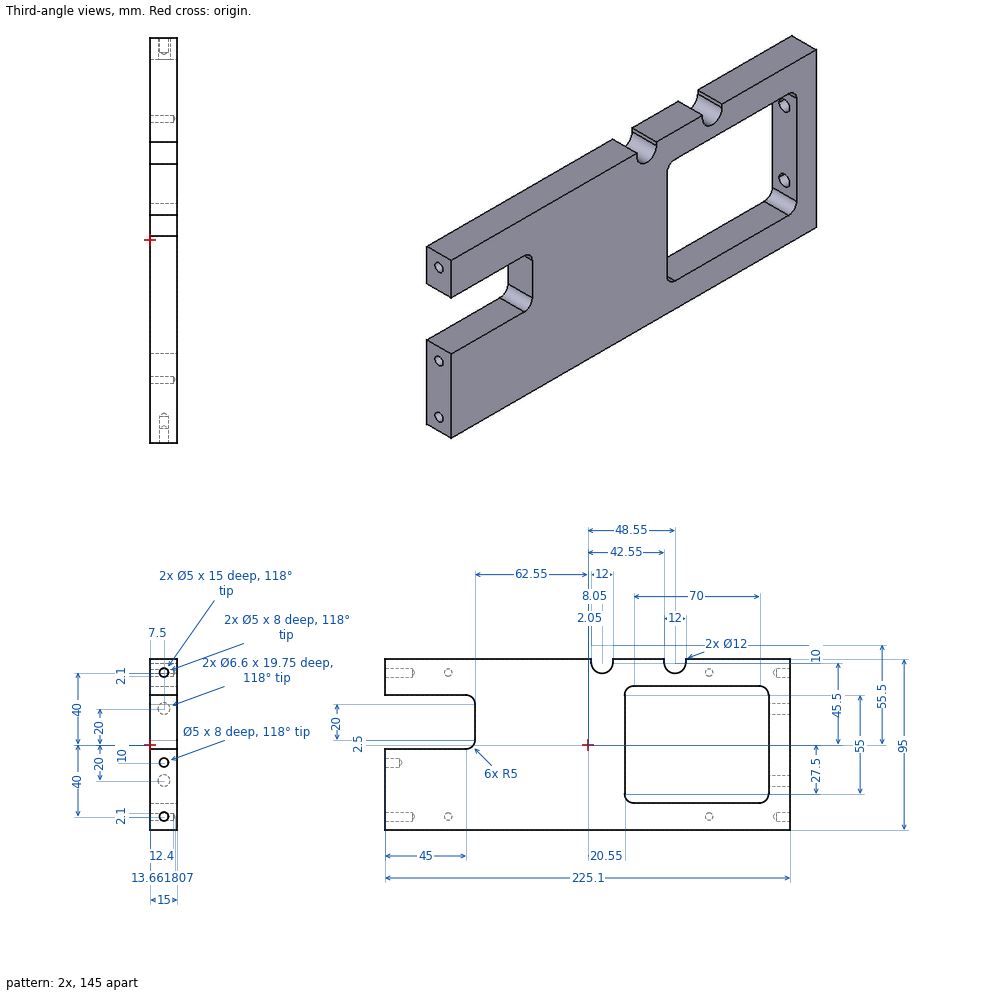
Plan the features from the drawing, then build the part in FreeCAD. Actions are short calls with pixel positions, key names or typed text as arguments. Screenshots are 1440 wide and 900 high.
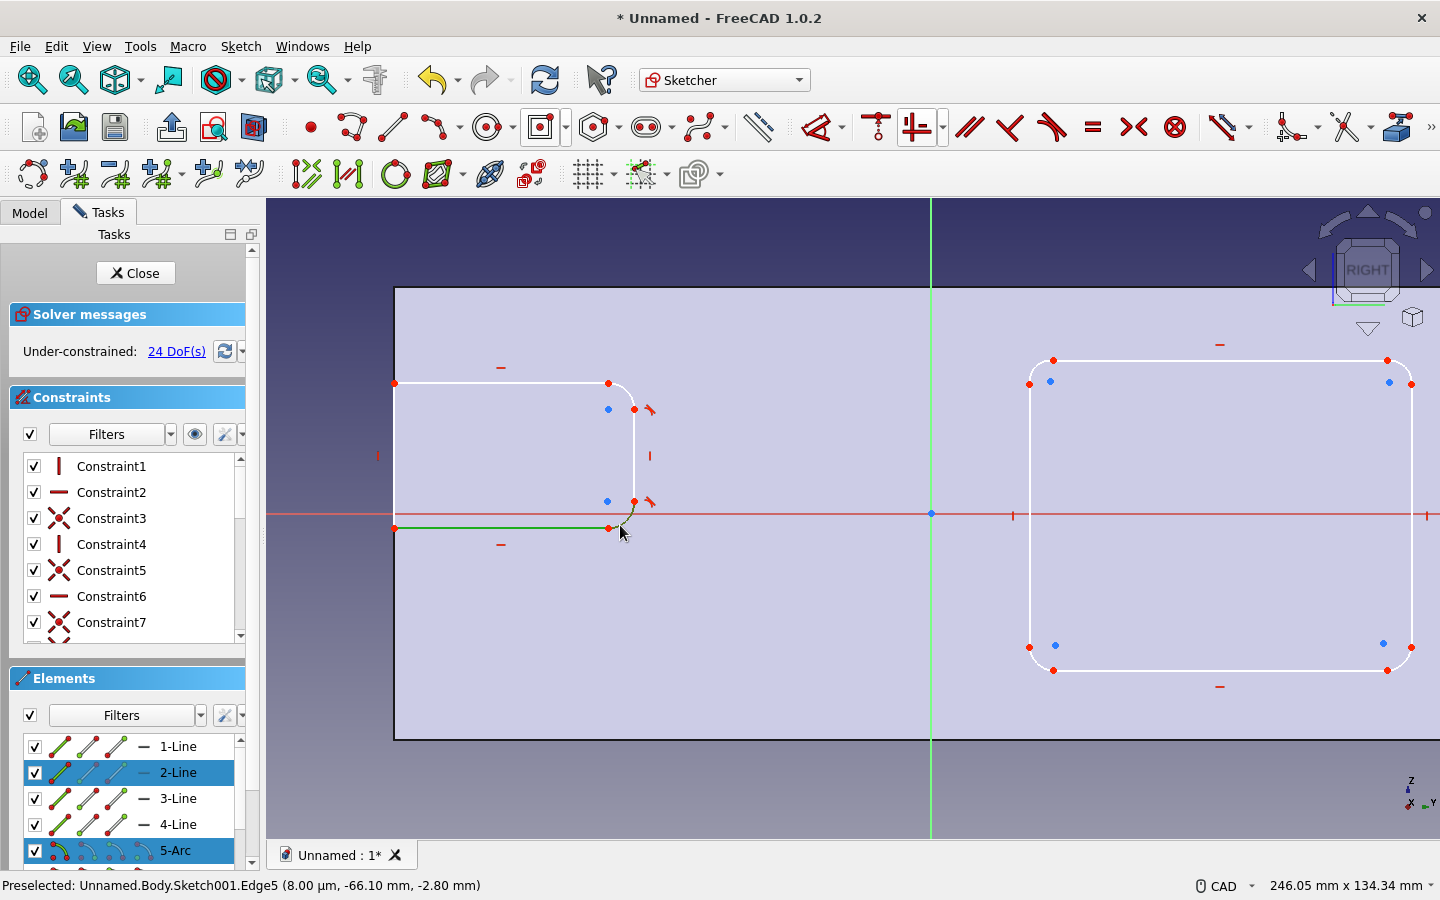
click(1052, 128)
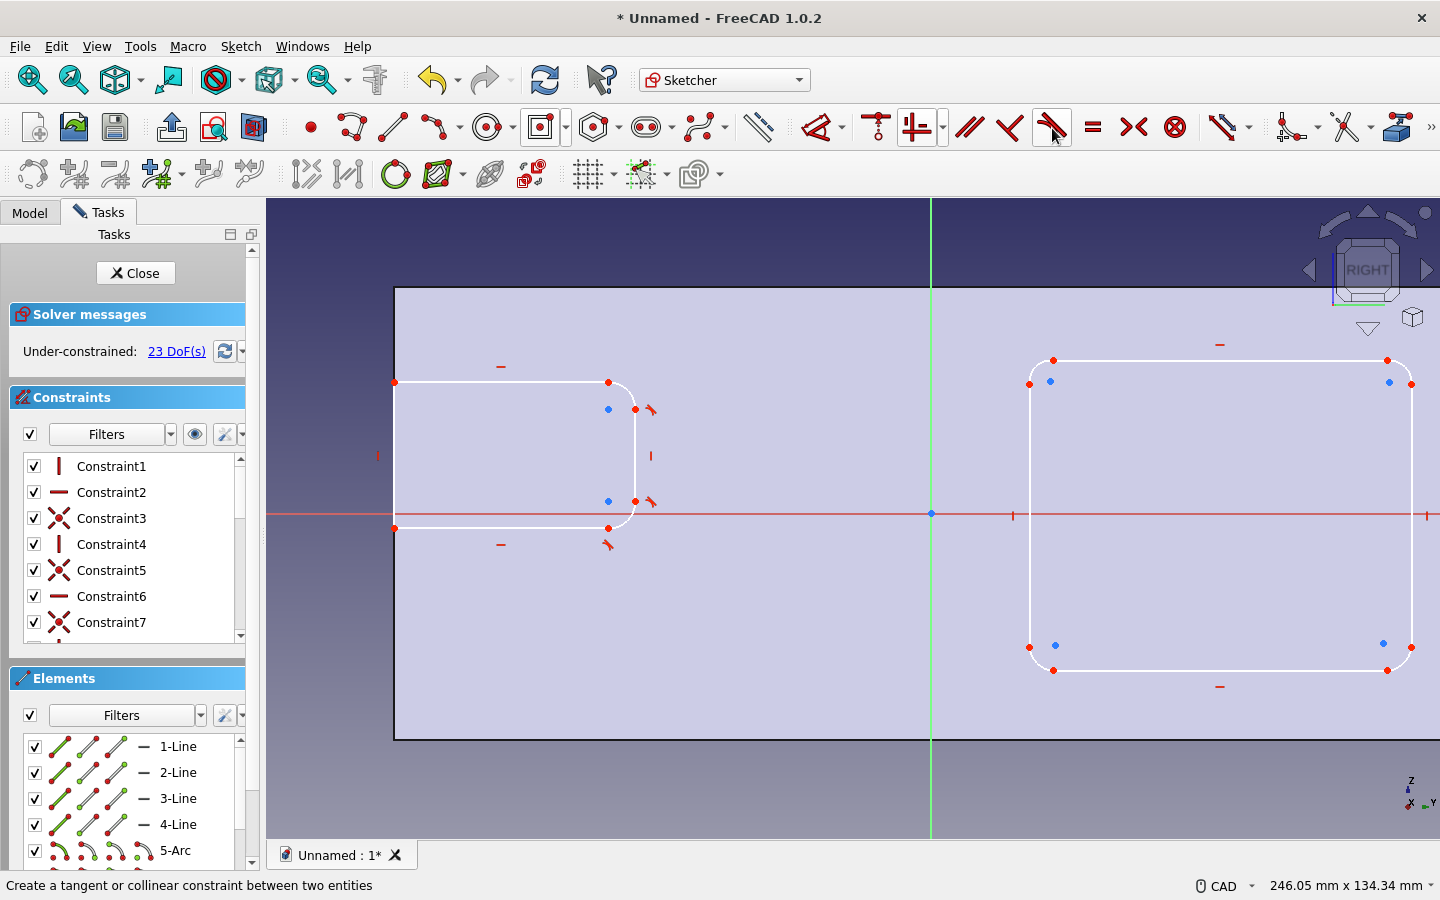
click(459, 382)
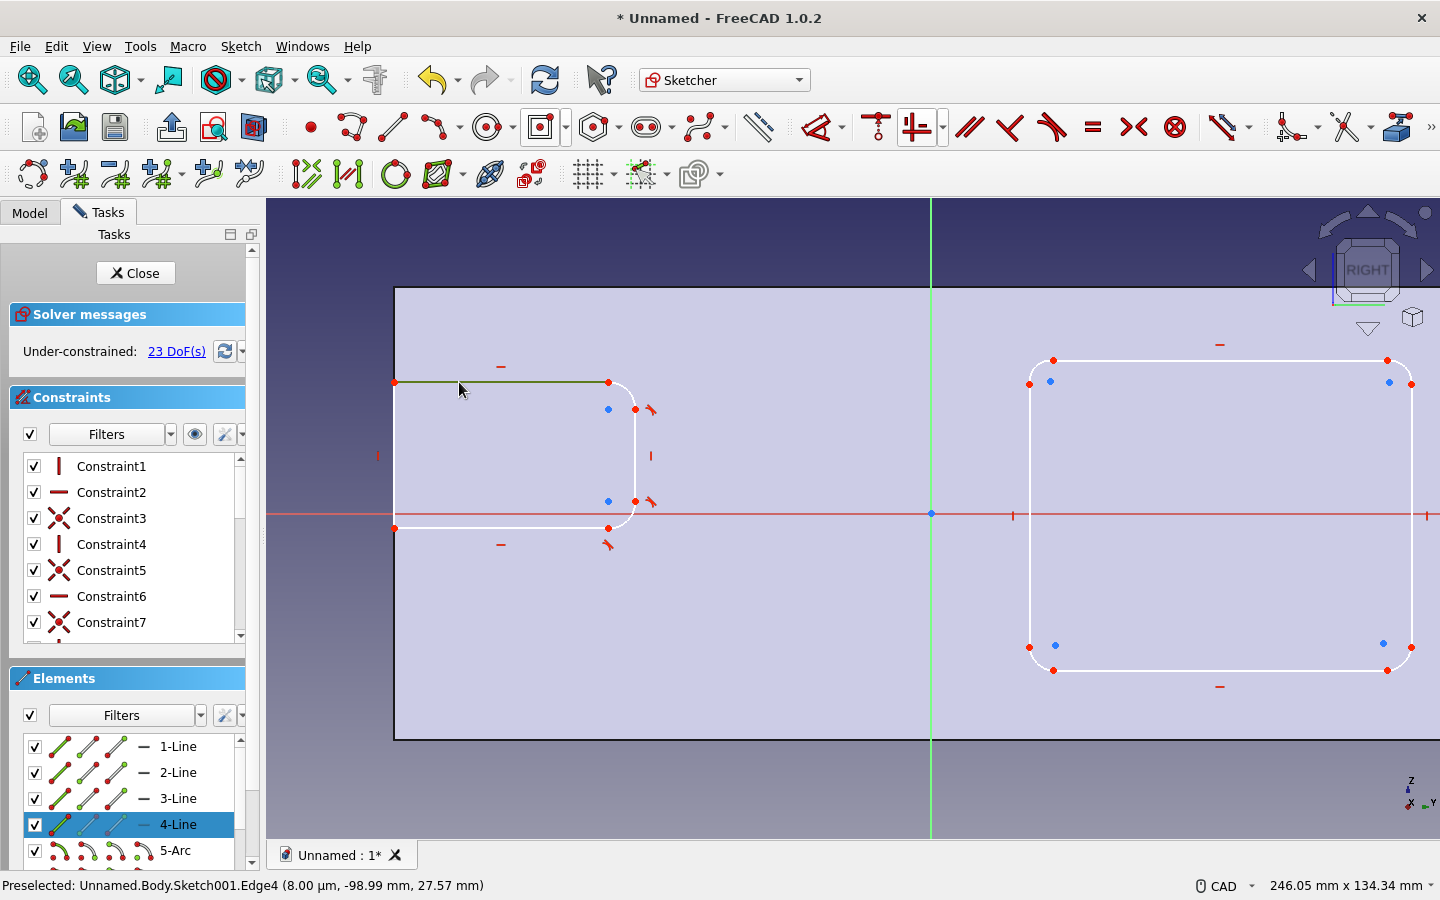
click(632, 397)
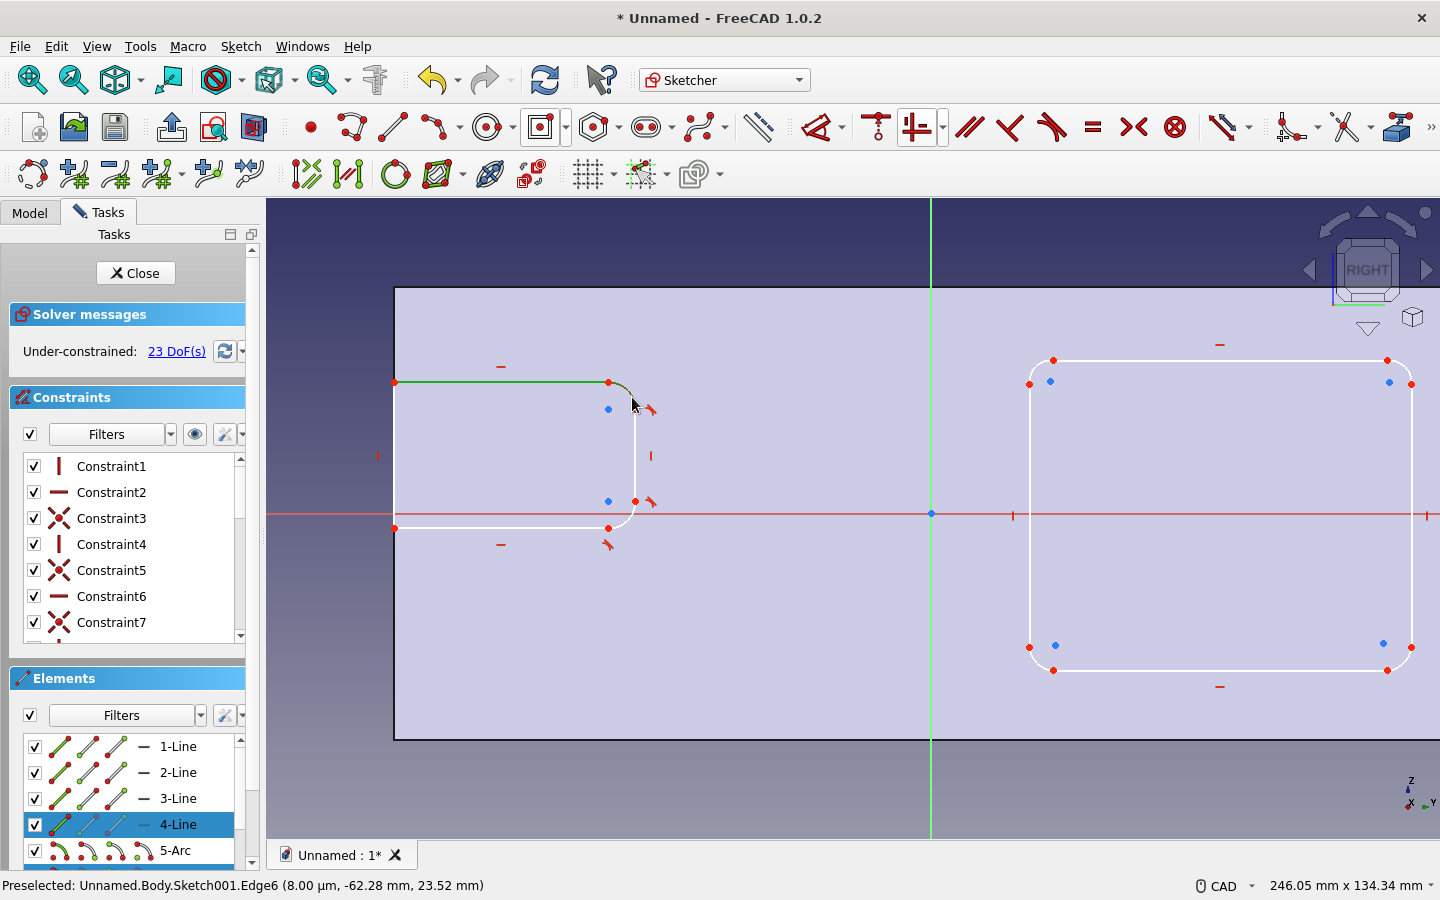
click(1052, 128)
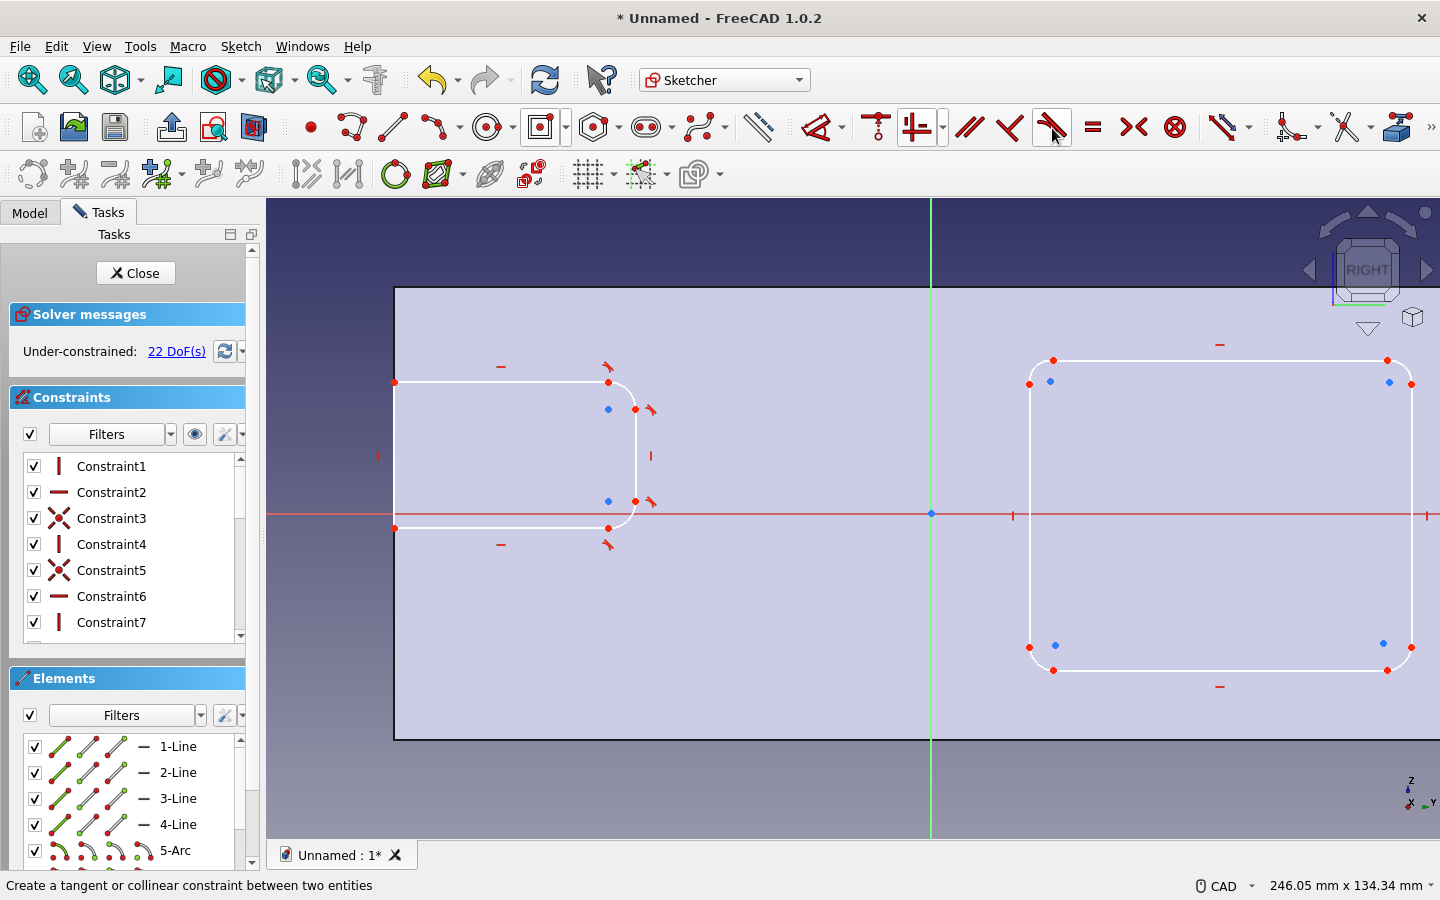
click(1030, 568)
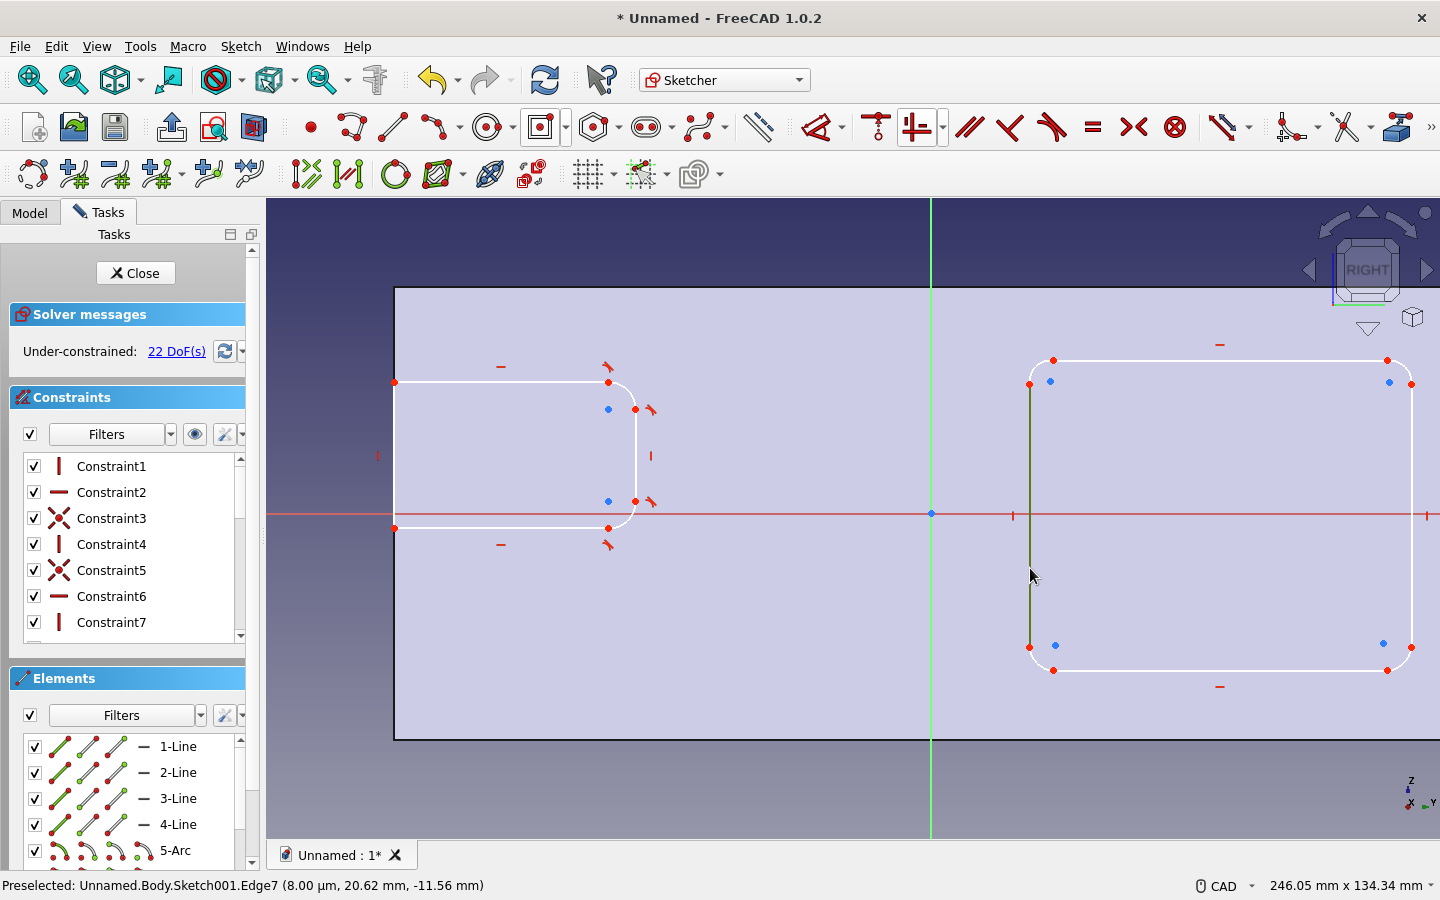
click(1042, 362)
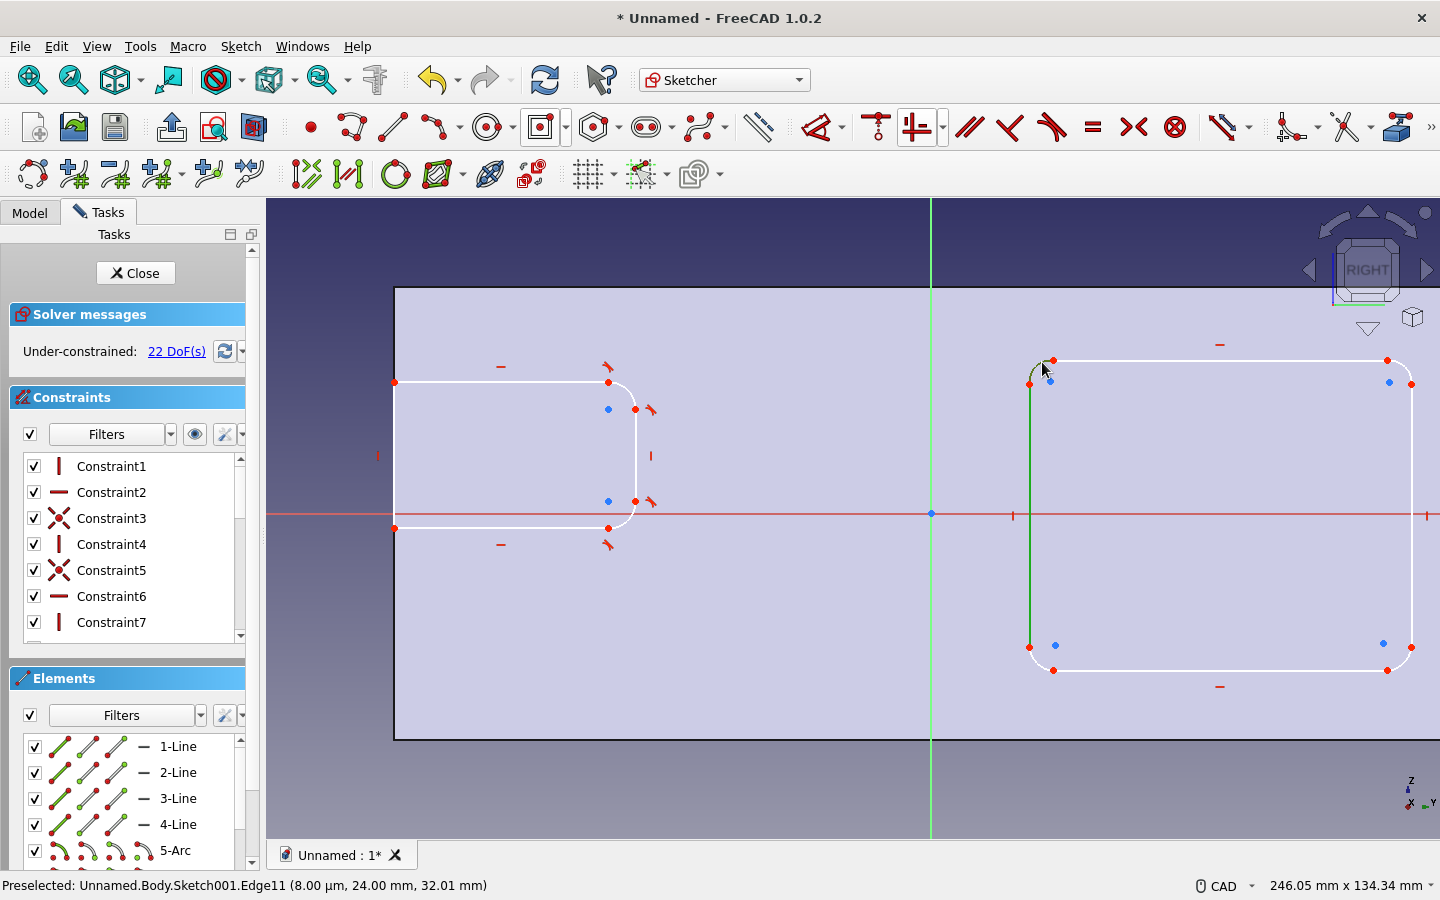
click(1052, 128)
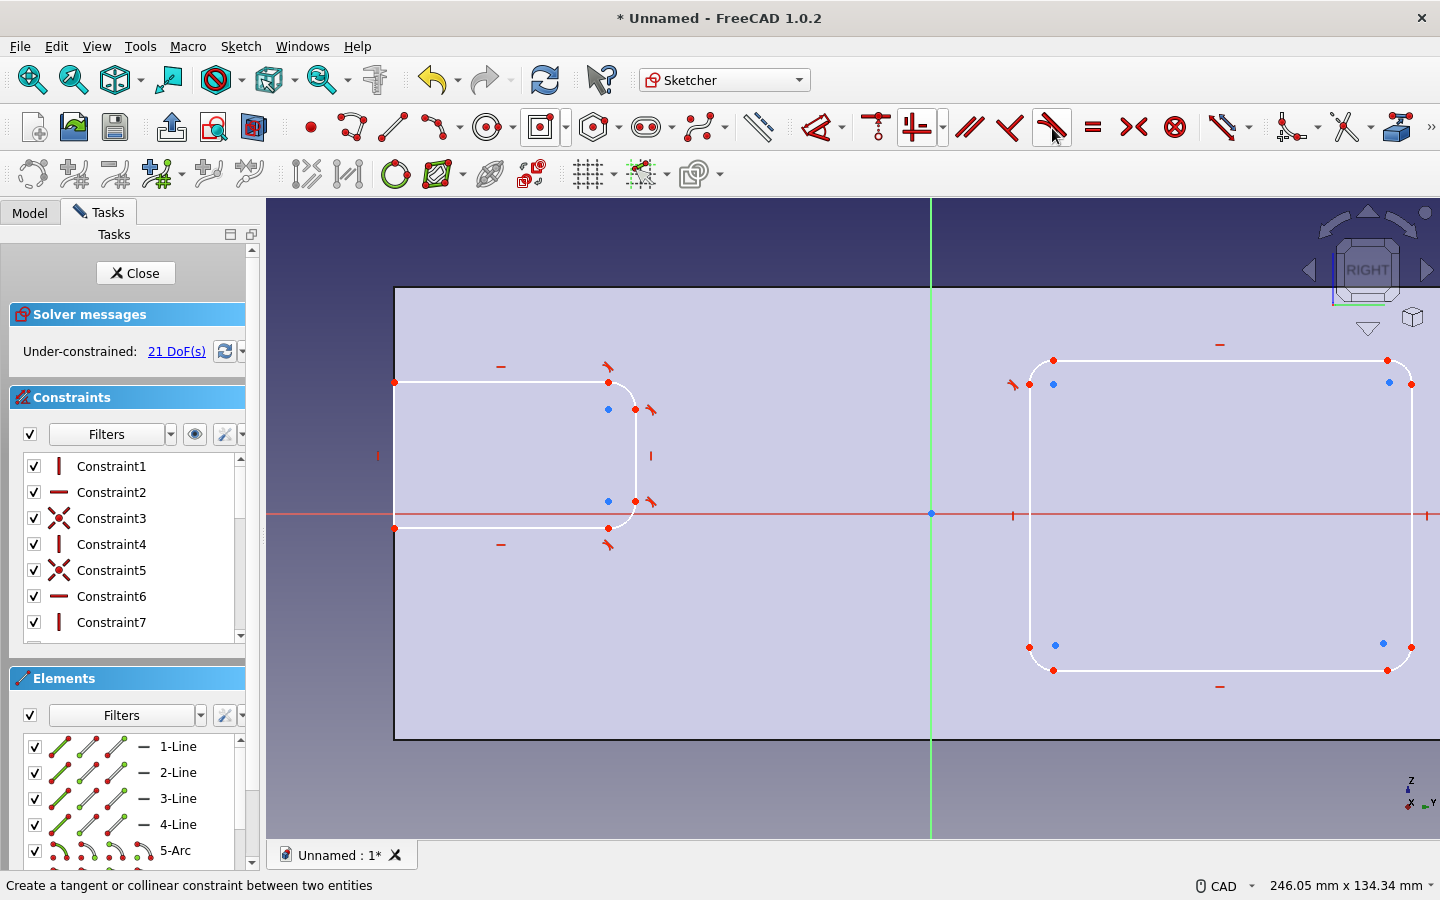
click(1030, 568)